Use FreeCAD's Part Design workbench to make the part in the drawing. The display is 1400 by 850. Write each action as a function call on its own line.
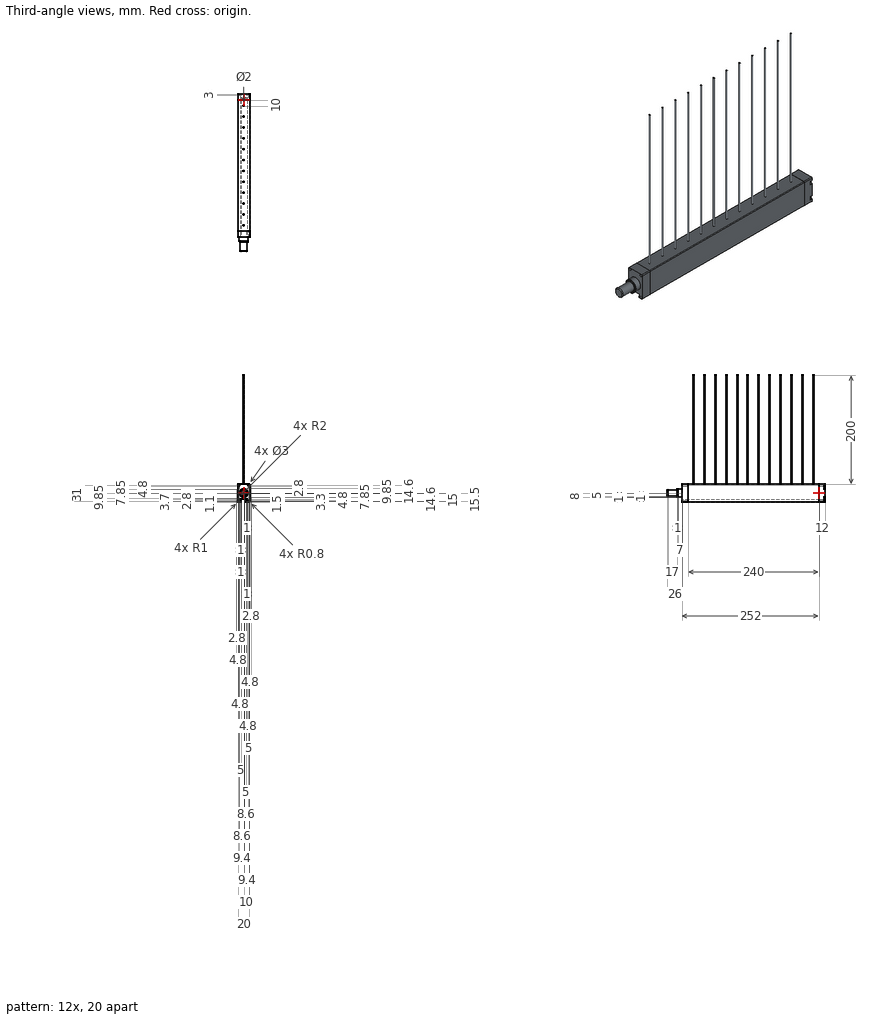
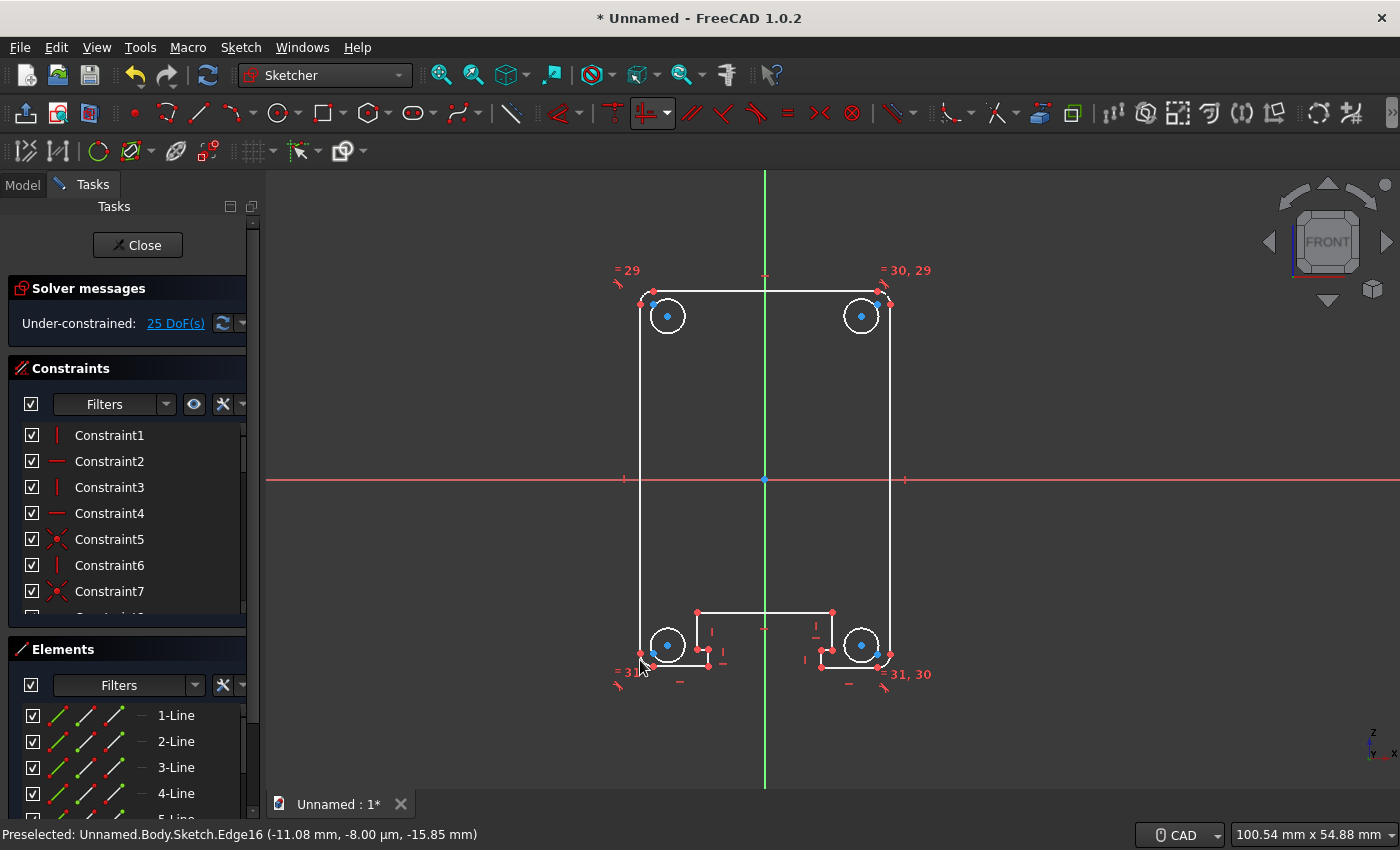
click(849, 304)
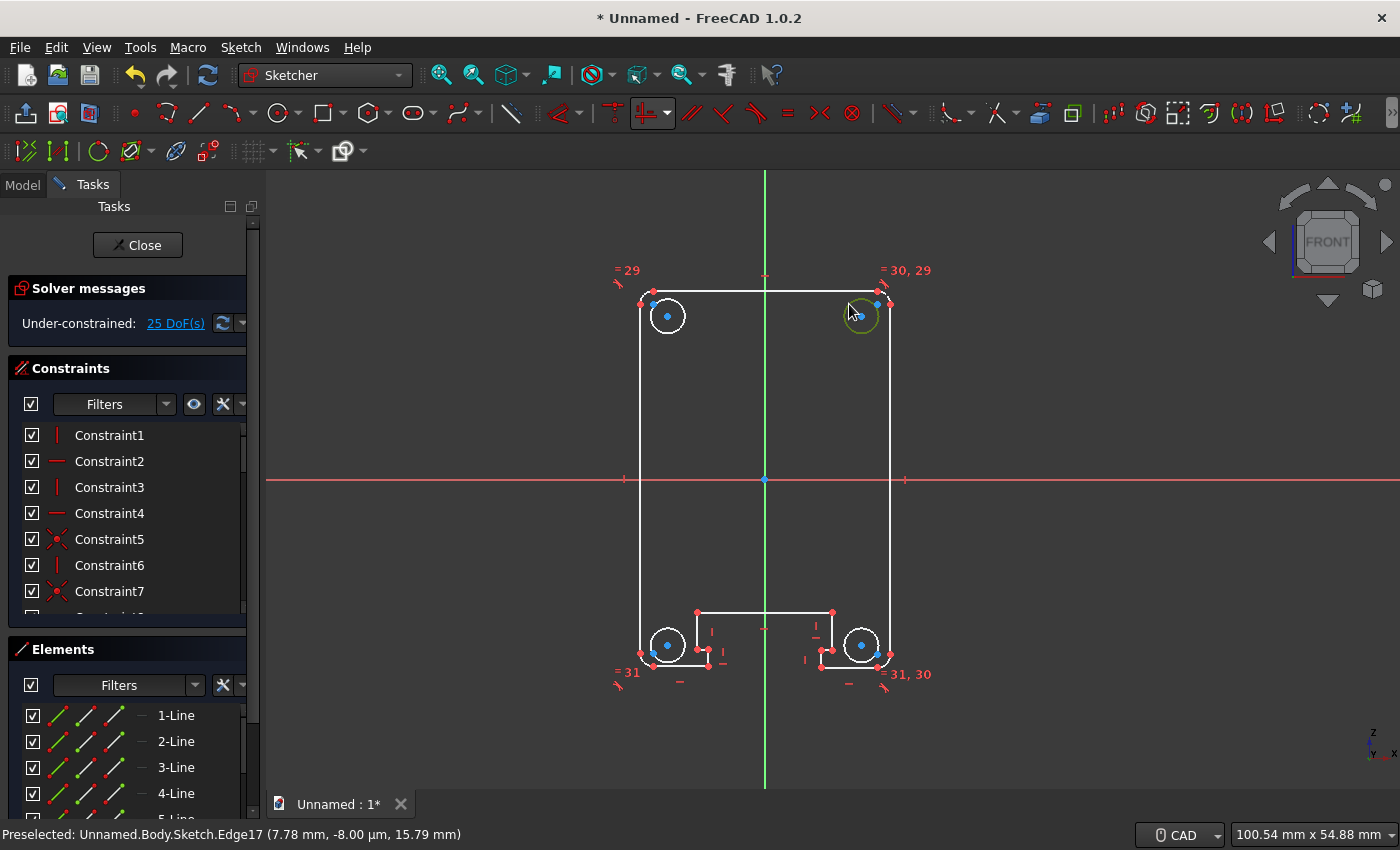
click(680, 304)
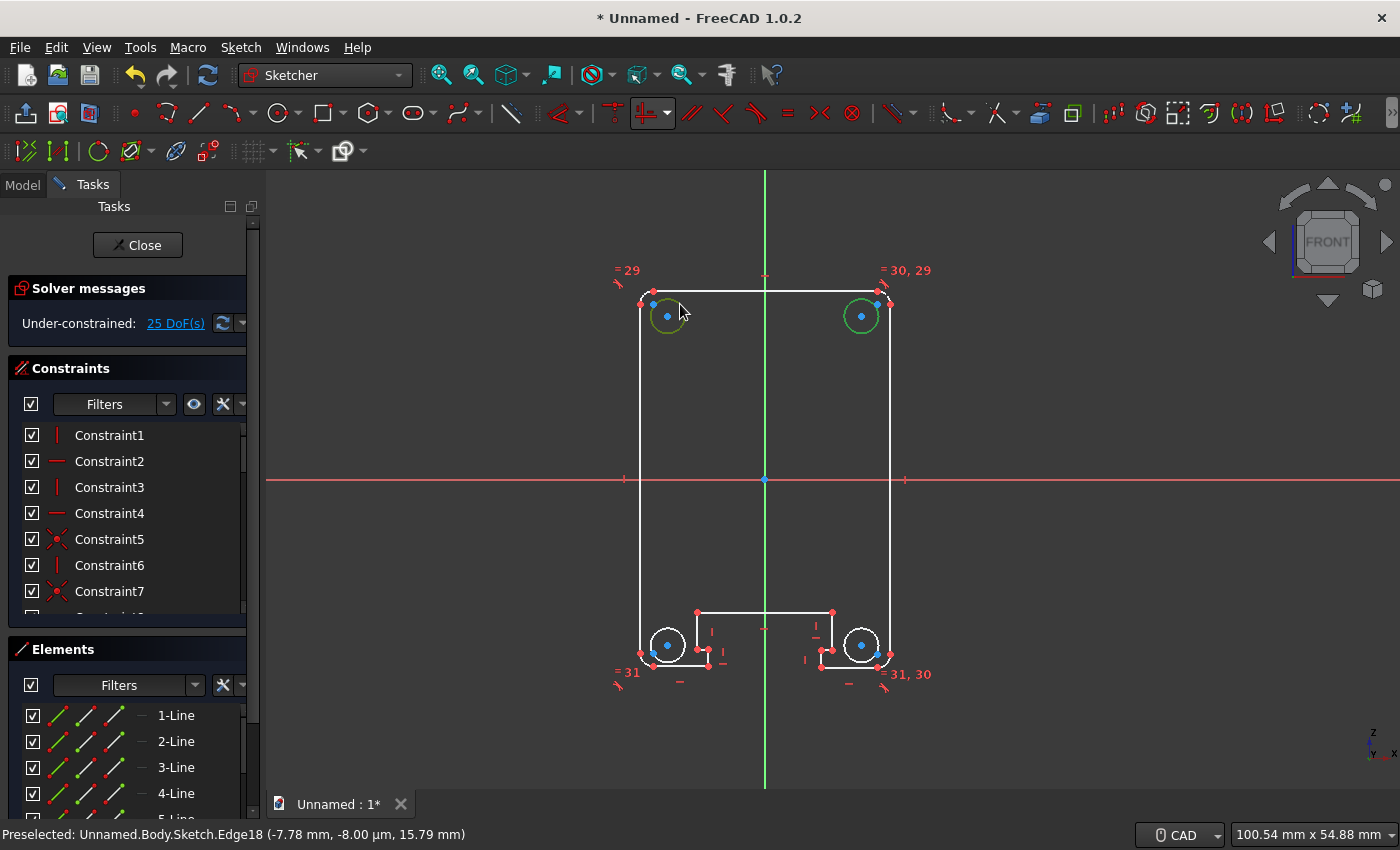
click(873, 633)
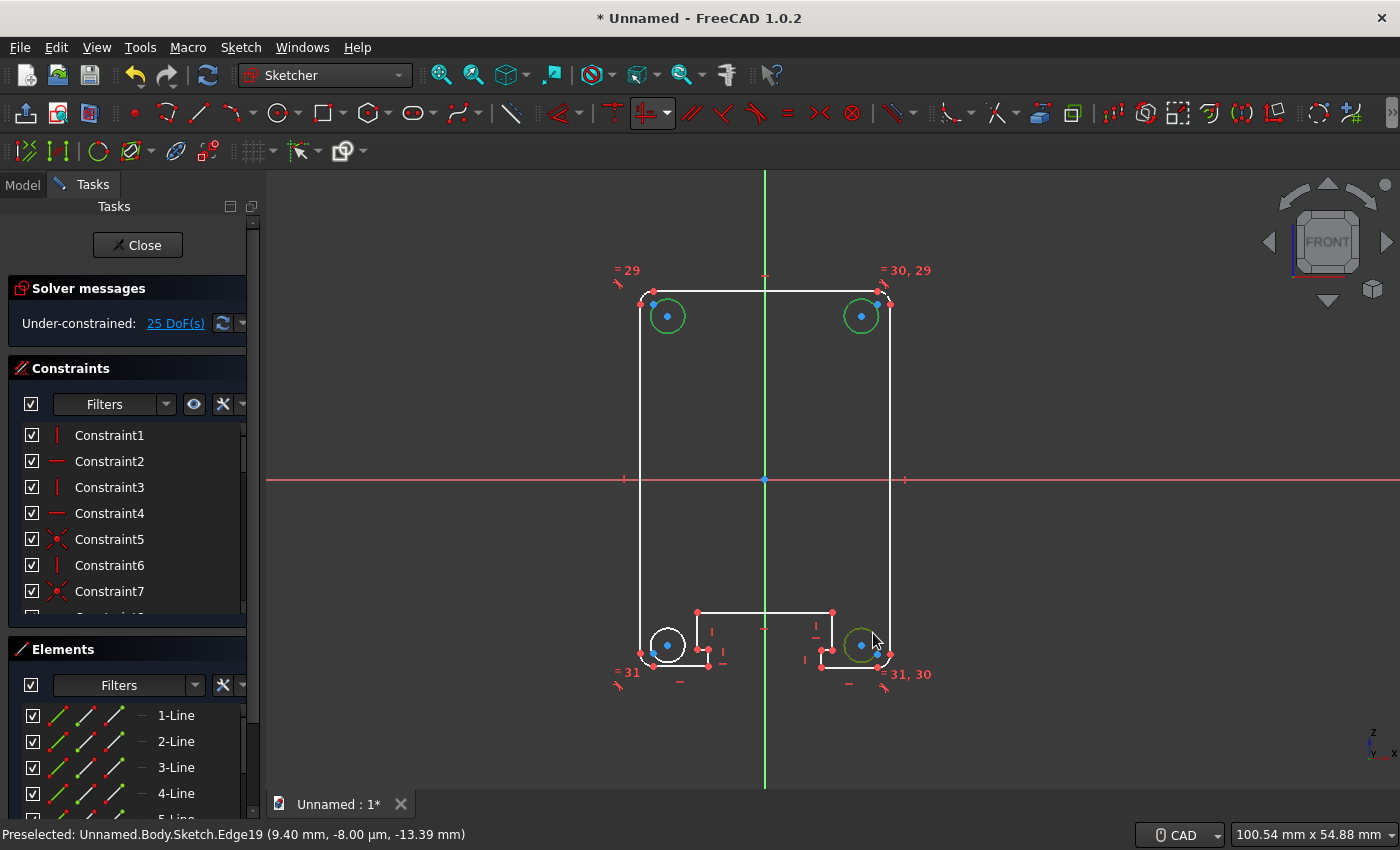
click(680, 633)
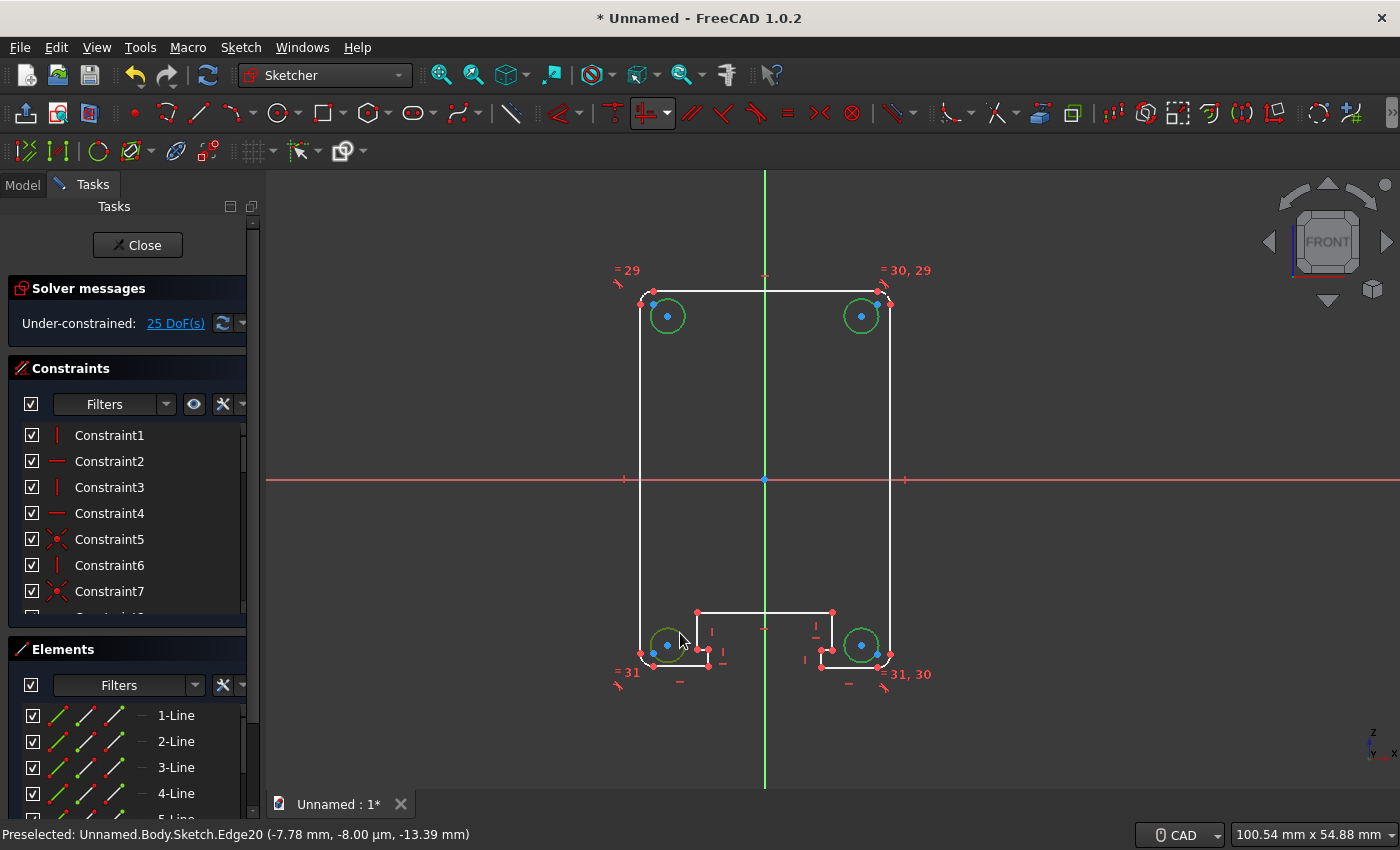
click(788, 114)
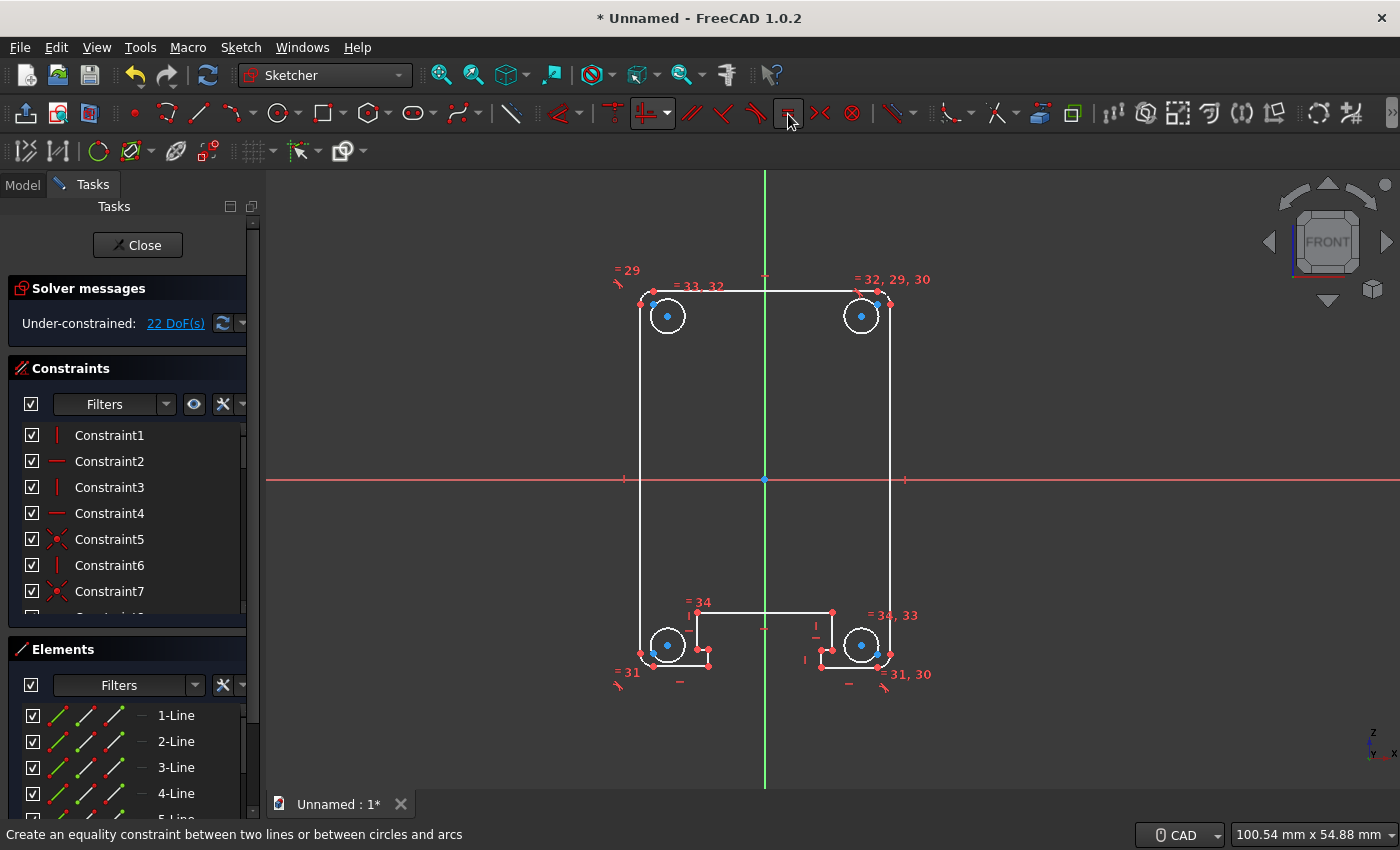
click(861, 316)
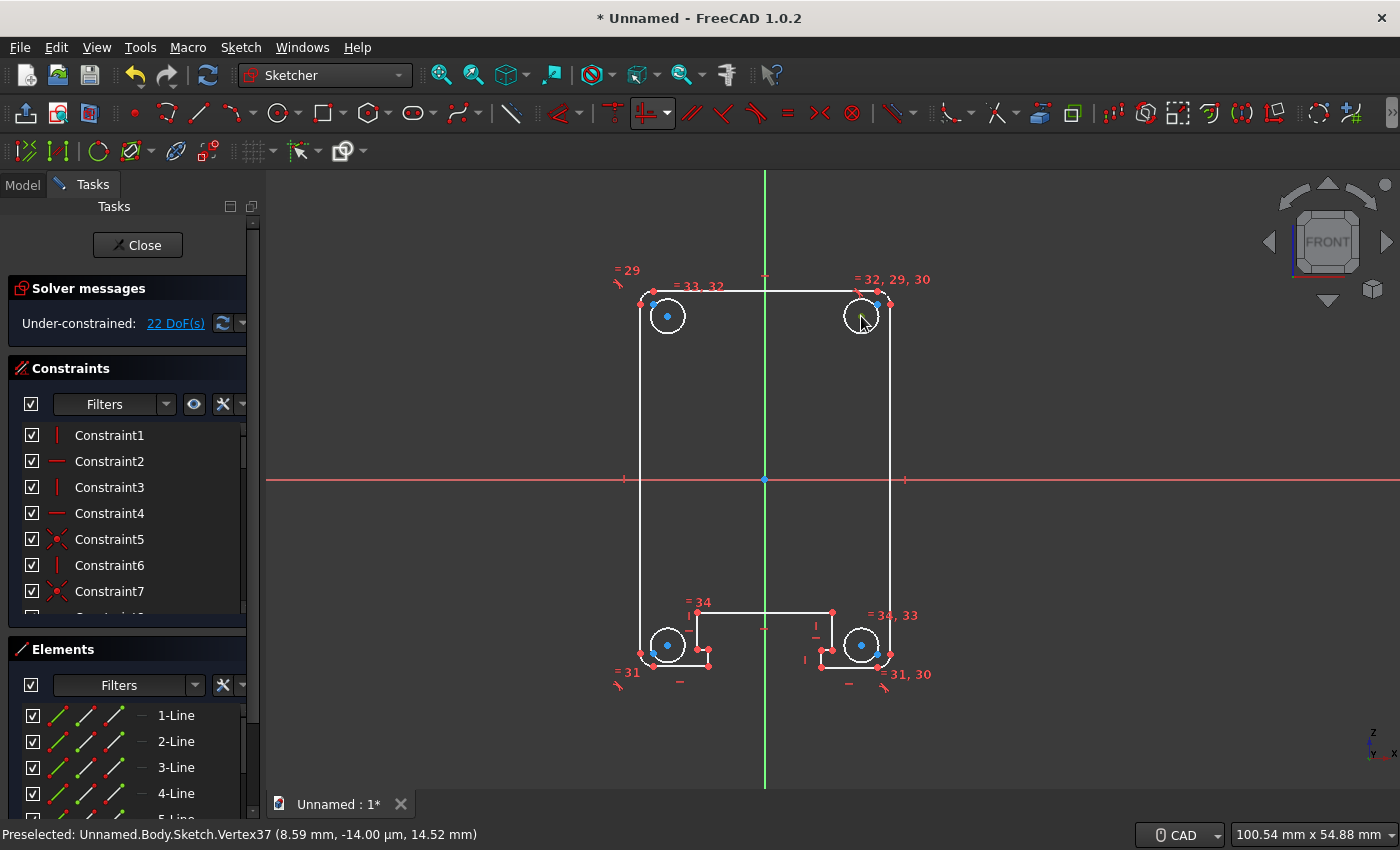
click(668, 316)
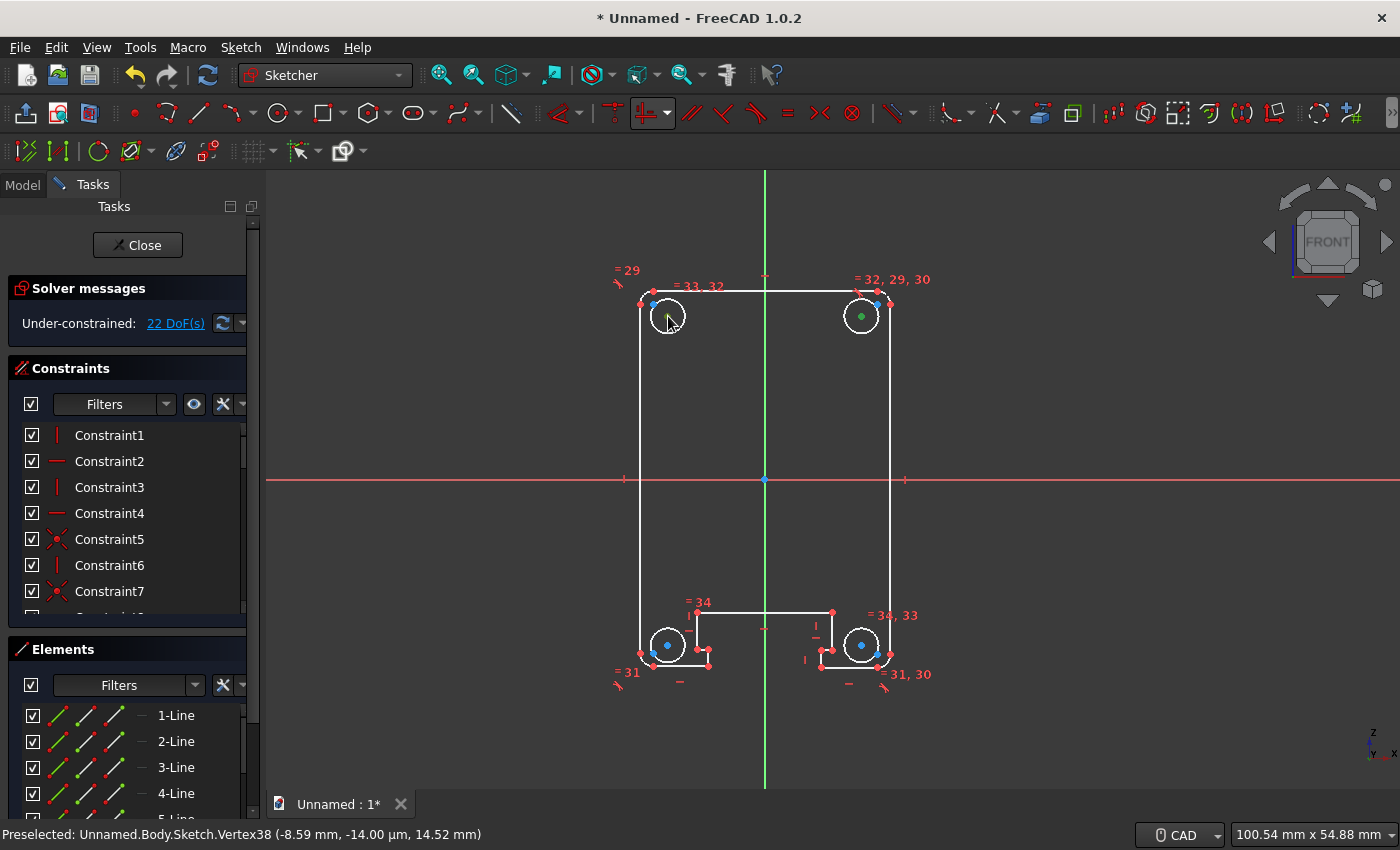
key(h)